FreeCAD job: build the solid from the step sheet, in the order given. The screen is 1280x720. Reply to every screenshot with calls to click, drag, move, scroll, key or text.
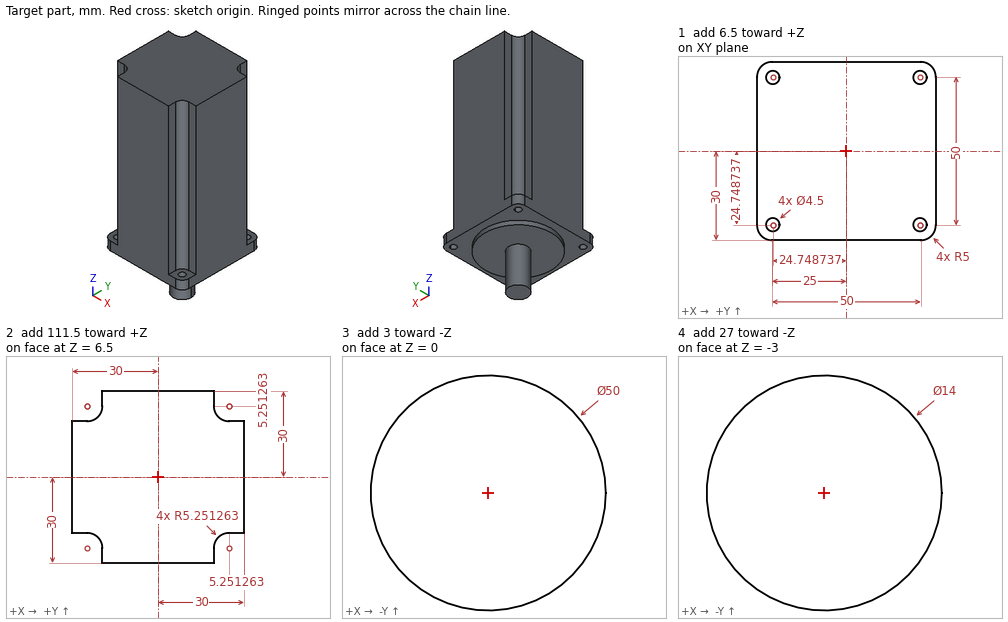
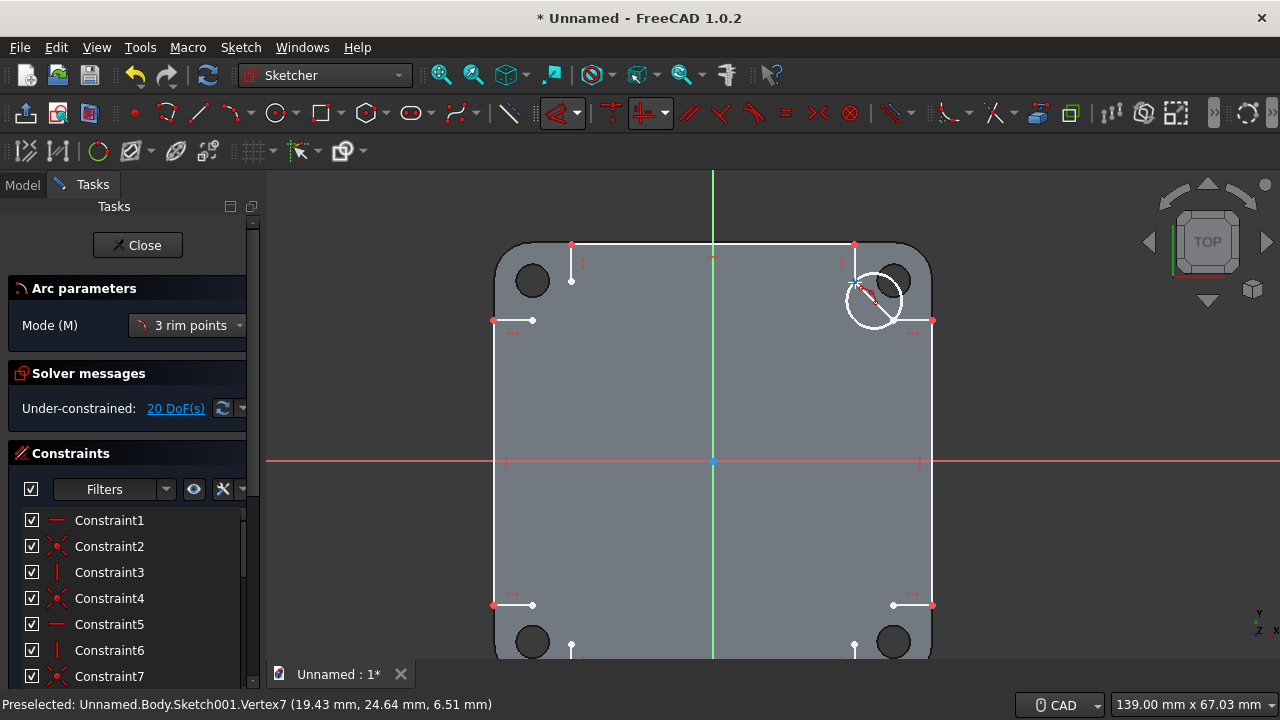
scroll(867, 308, up, 2)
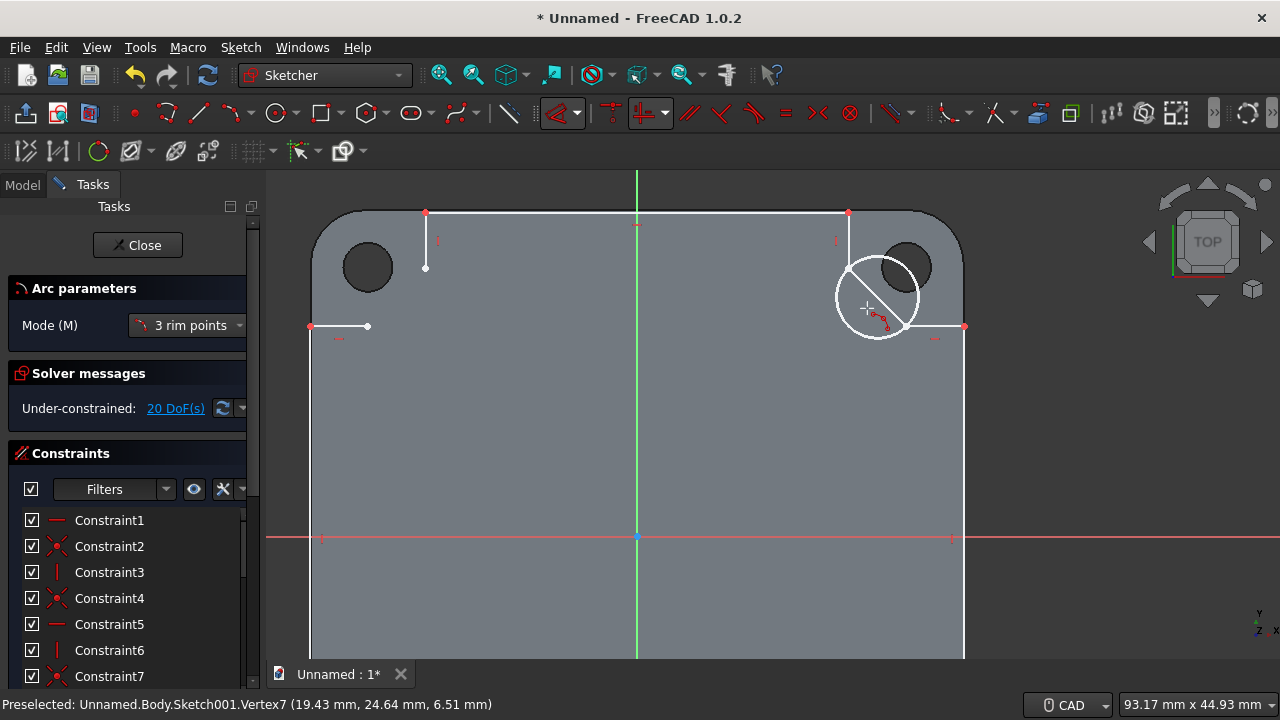
click(866, 308)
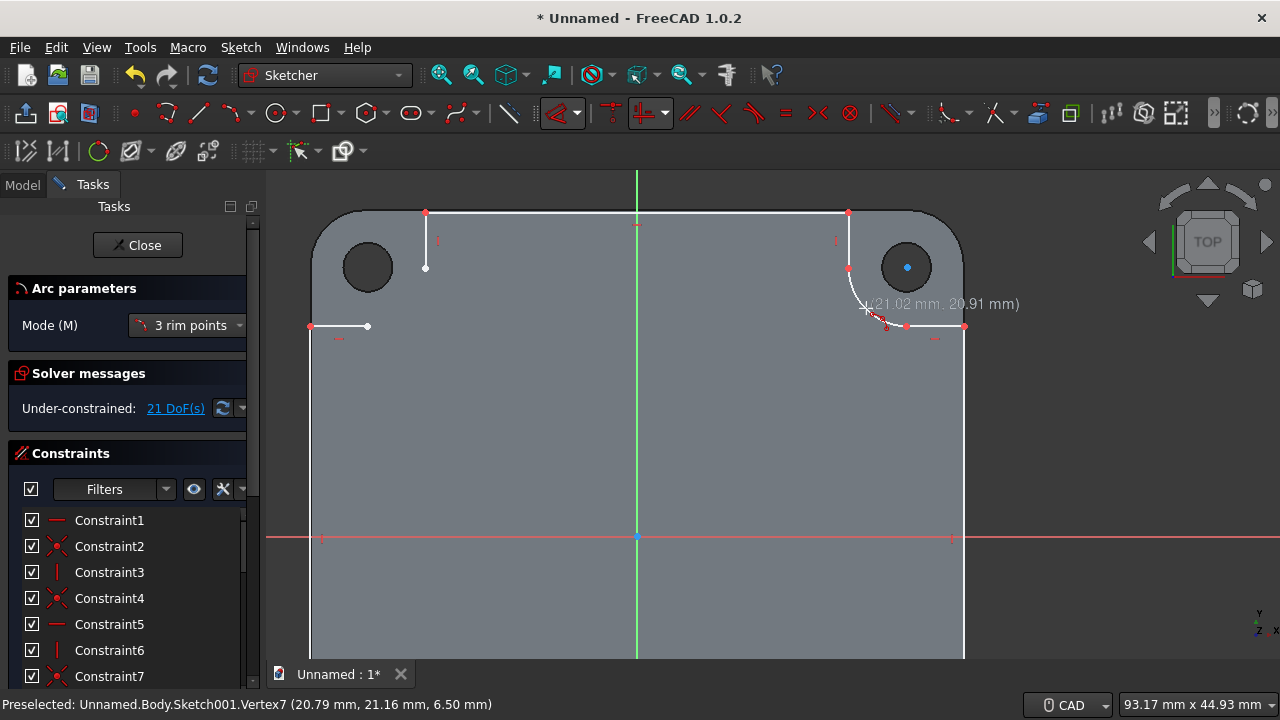
click(426, 268)
click(368, 326)
click(408, 308)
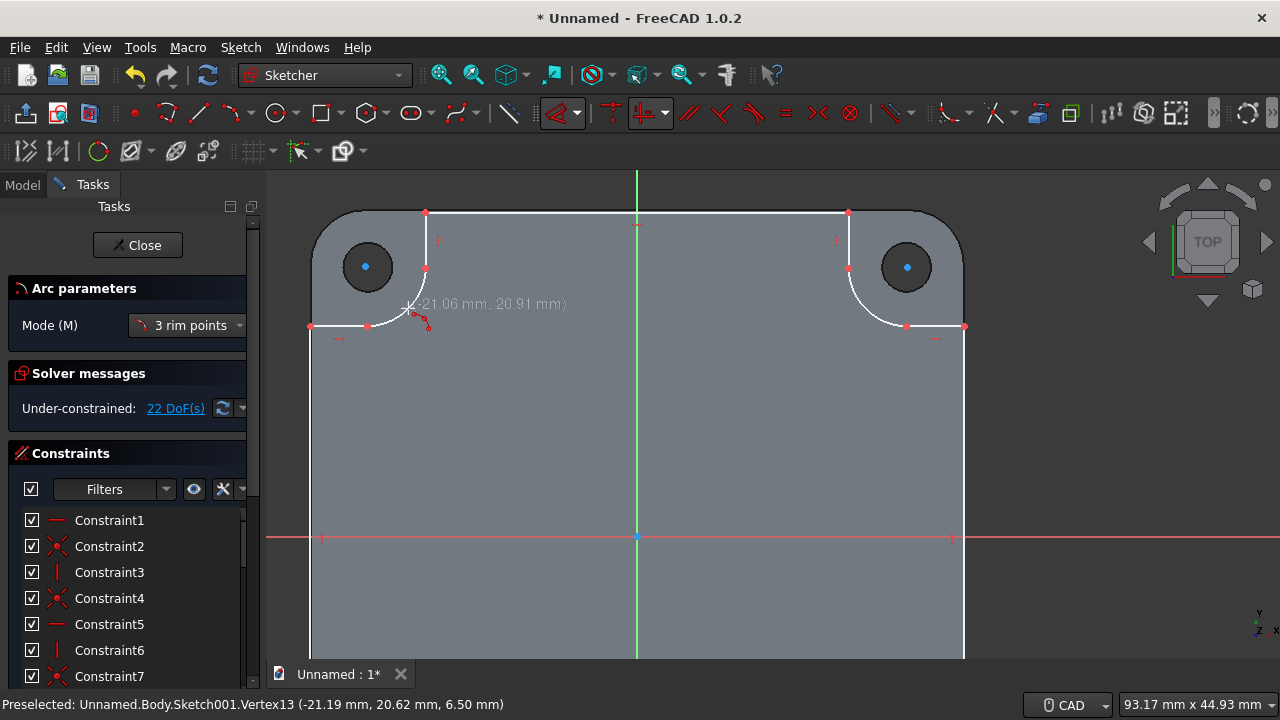
scroll(759, 315, down, 4)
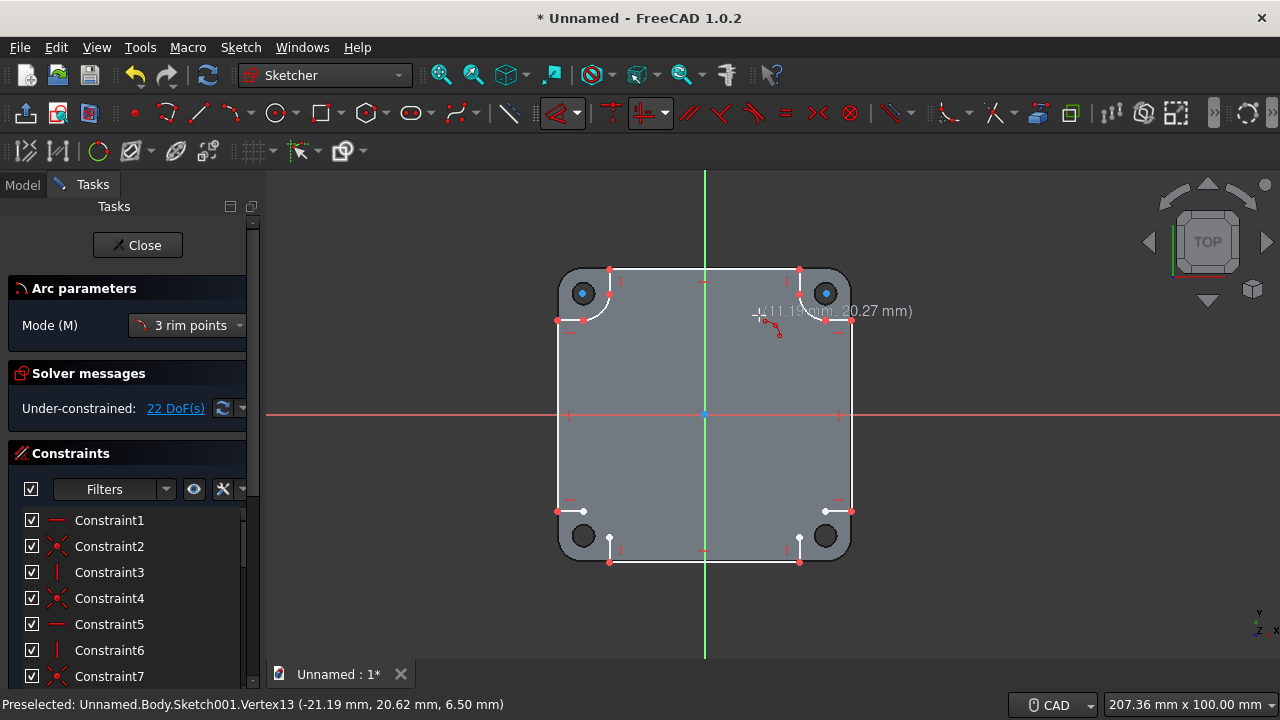
scroll(584, 510, up, 2)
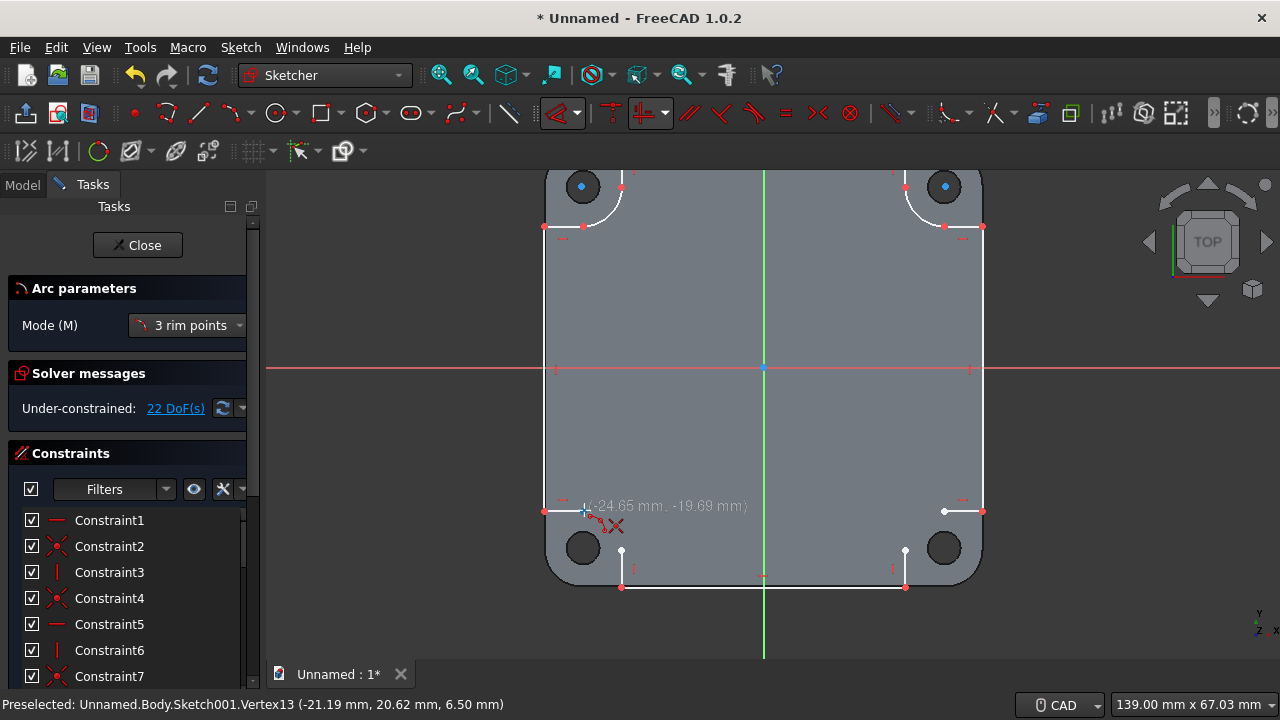
click(583, 511)
click(622, 550)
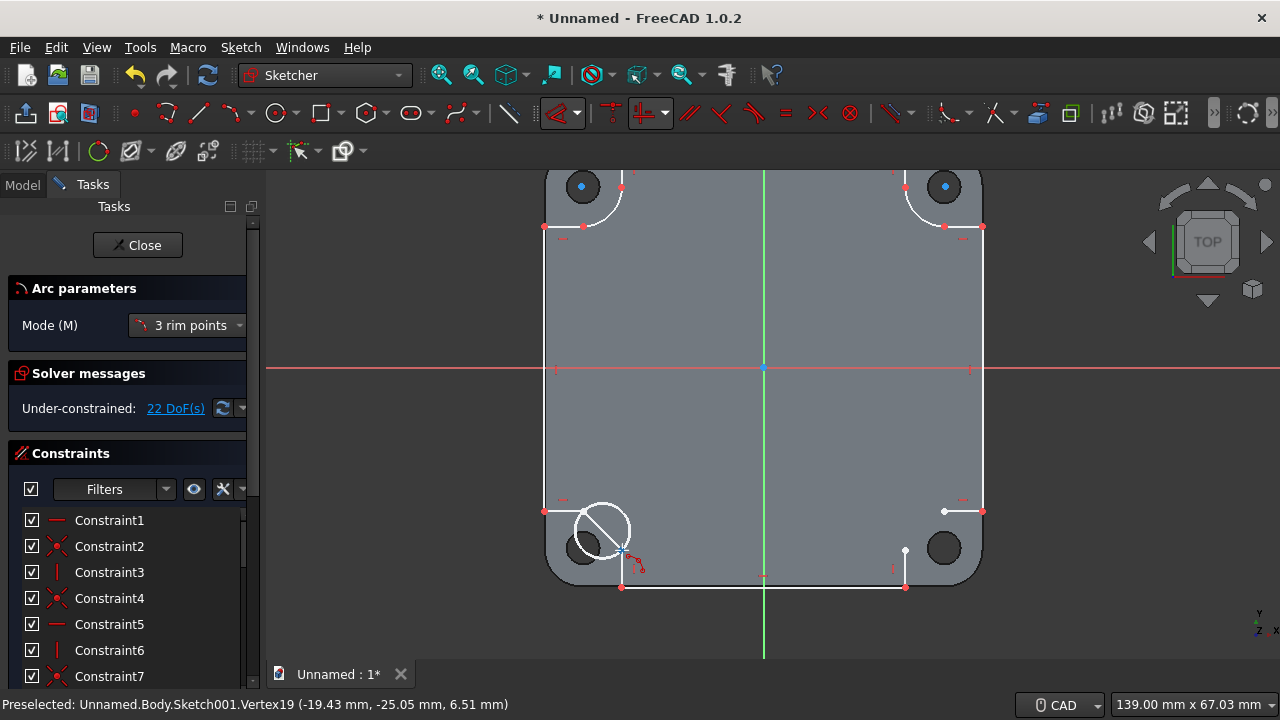
scroll(610, 521, up, 2)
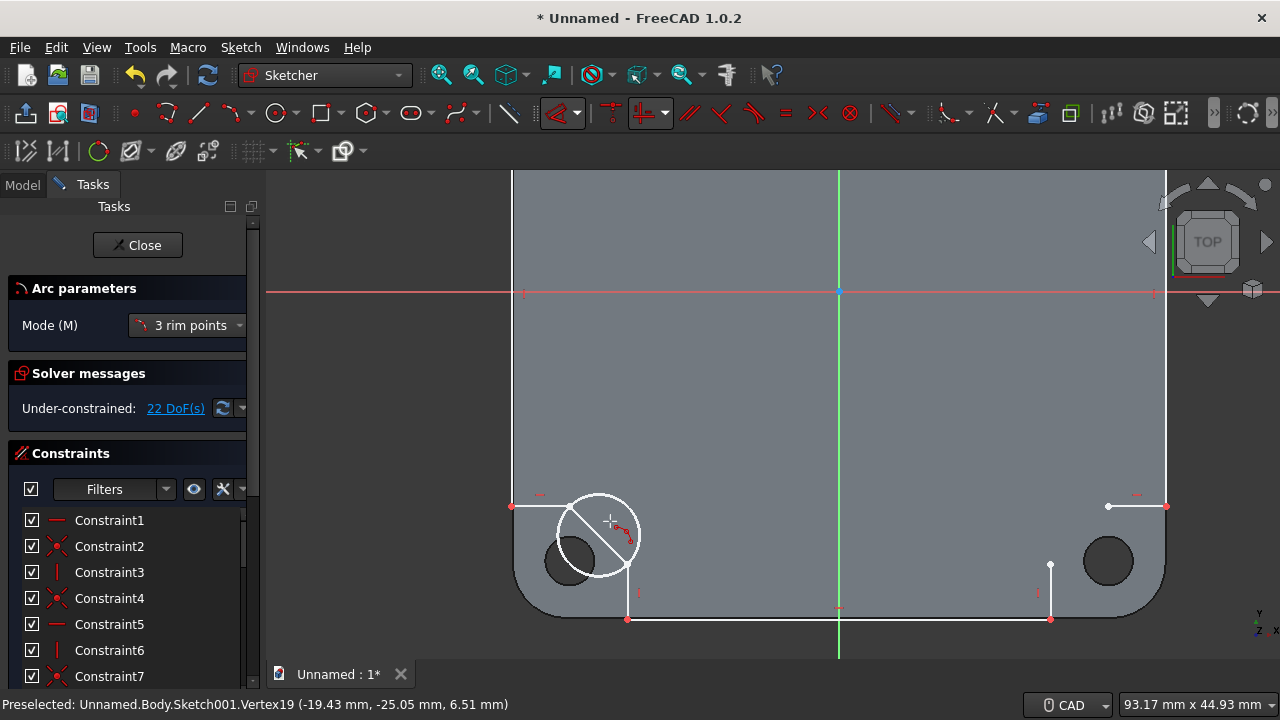
click(610, 521)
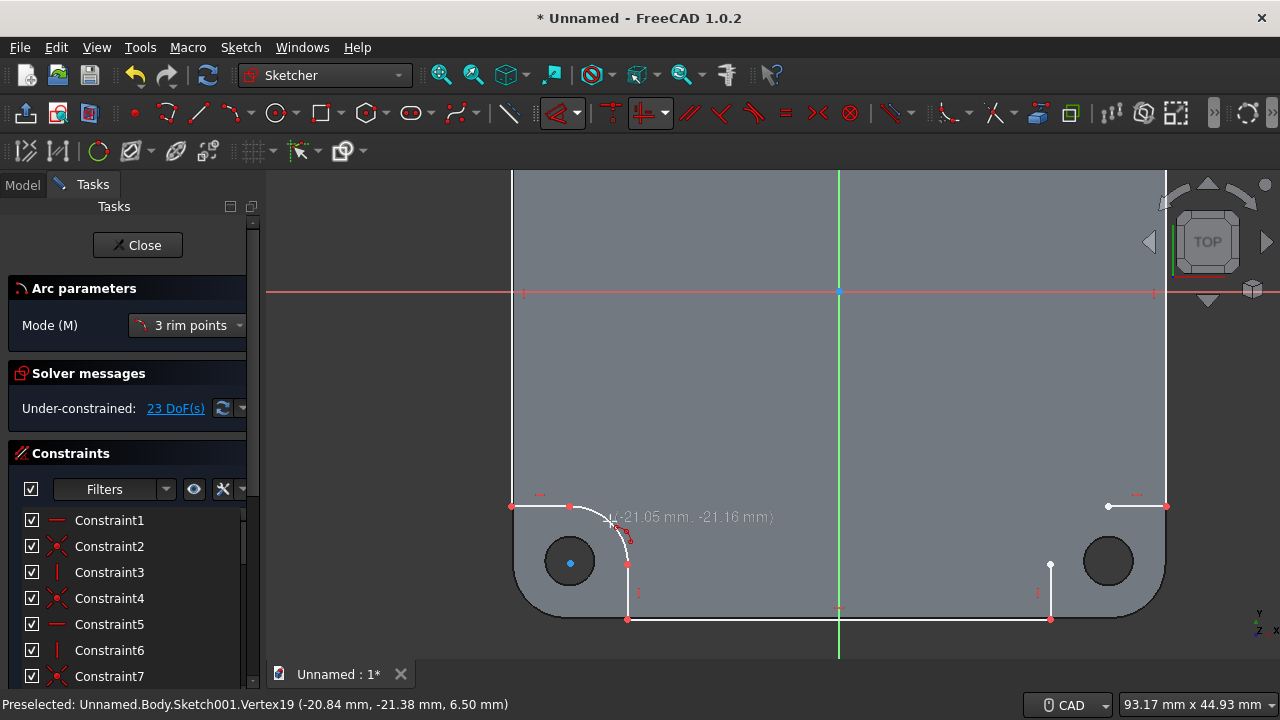
click(1051, 564)
click(1108, 506)
click(1068, 521)
key(Escape)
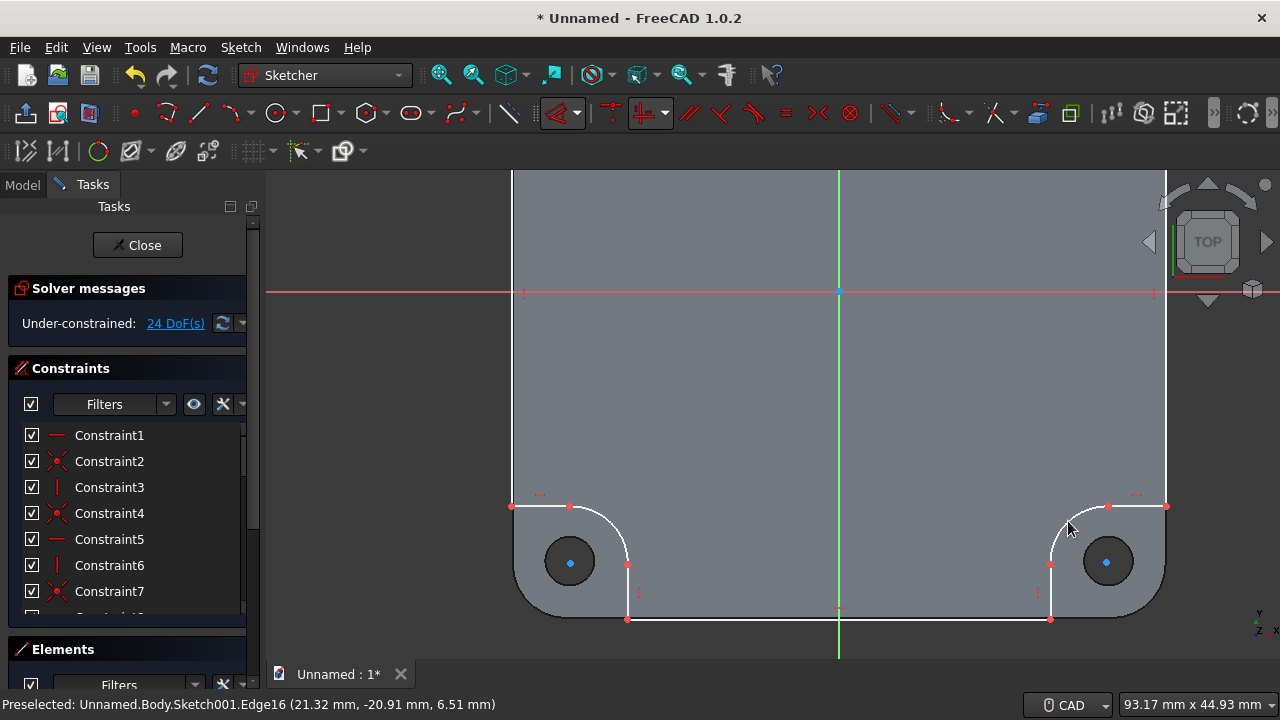
scroll(595, 515, down, 4)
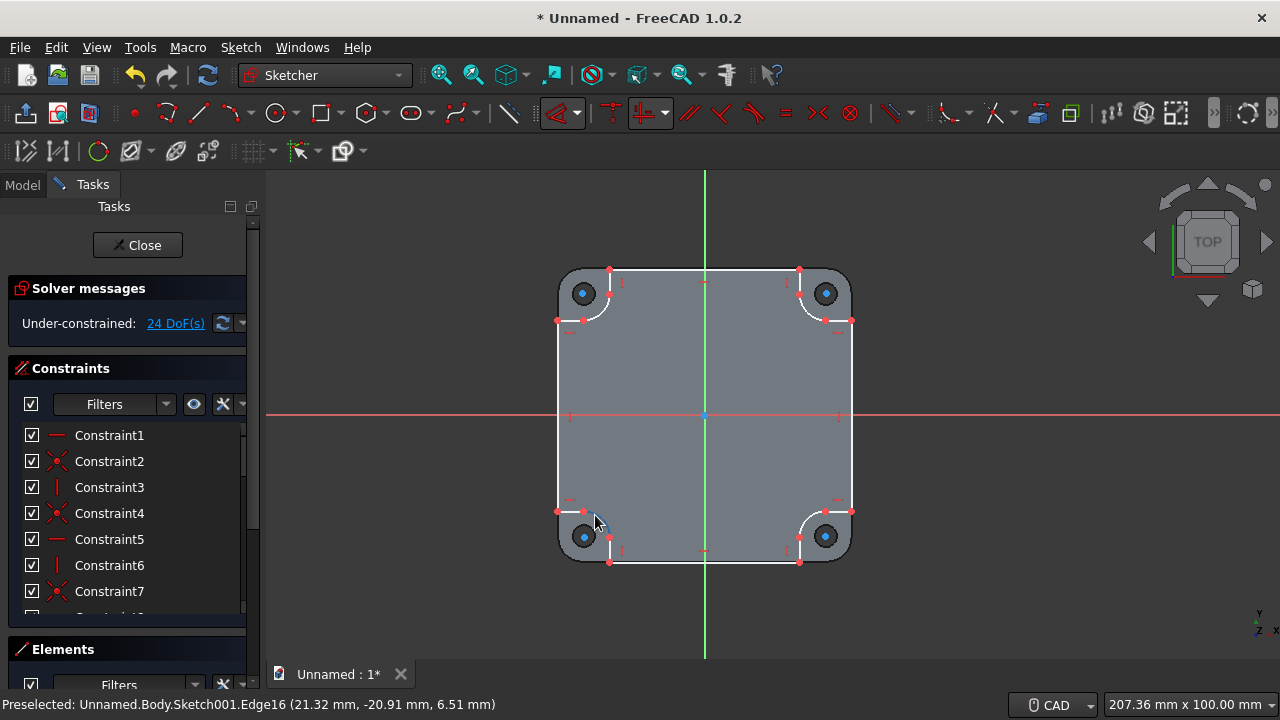
scroll(834, 512, up, 3)